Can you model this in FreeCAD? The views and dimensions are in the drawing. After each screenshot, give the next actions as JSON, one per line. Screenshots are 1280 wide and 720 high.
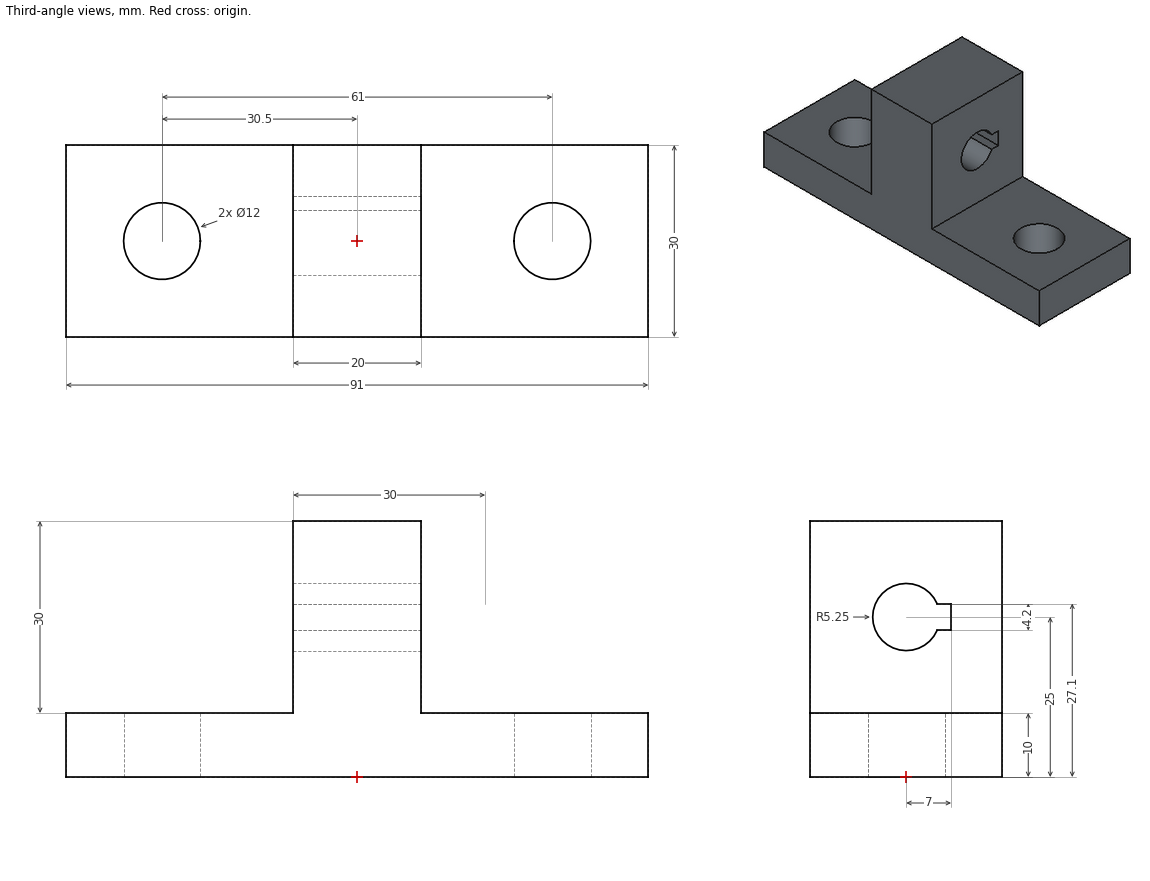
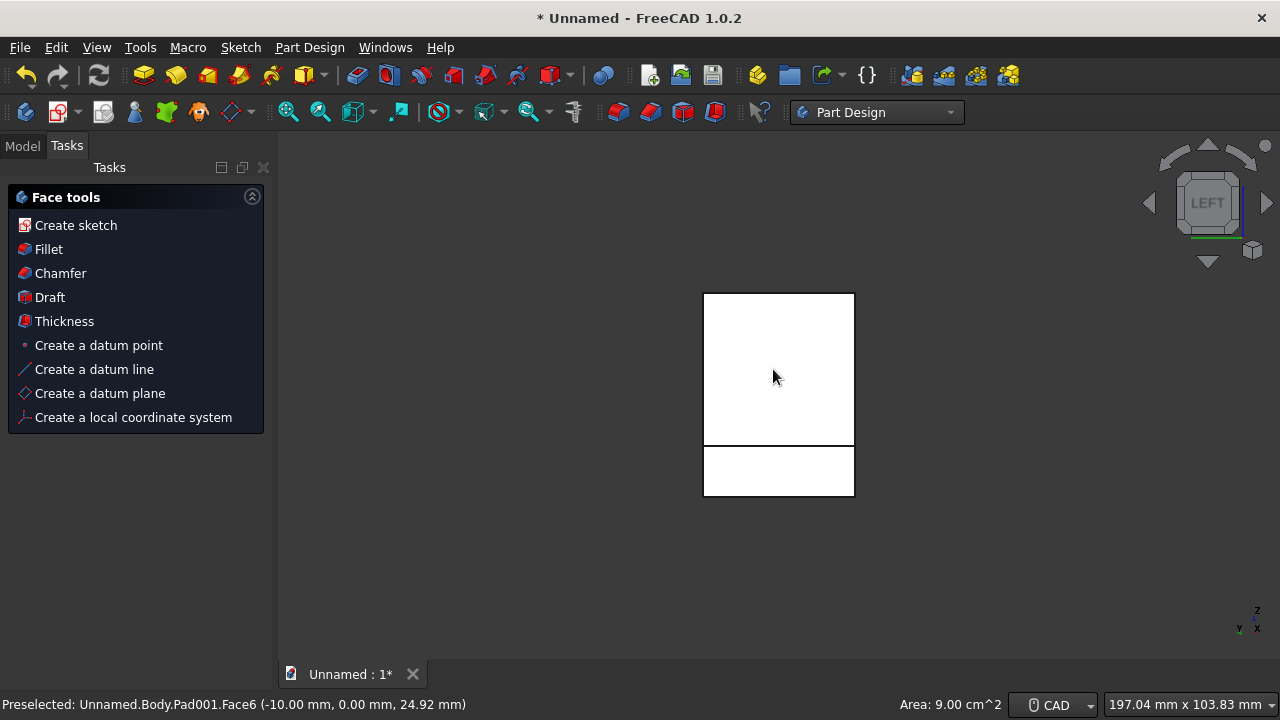
{"action": "left_click", "coordinate": [58, 112]}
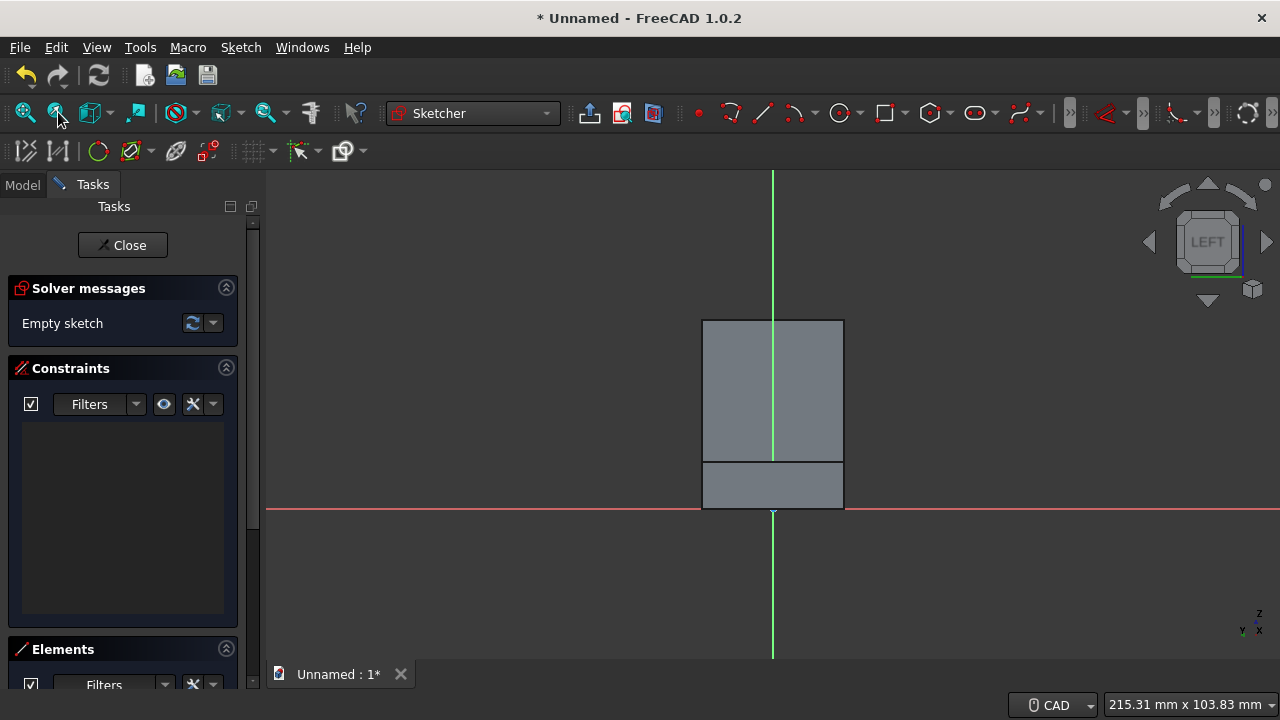
{"action": "key", "text": "q s"}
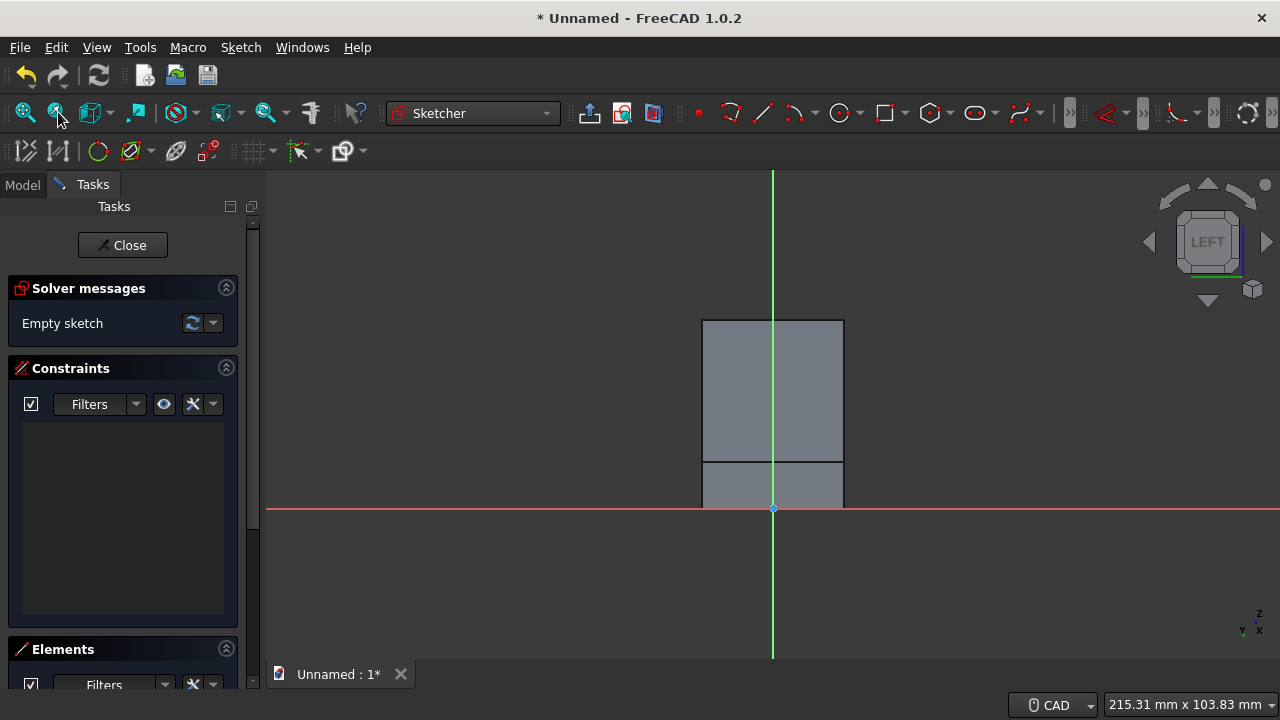
{"action": "scroll", "coordinate": [821, 470], "scroll_direction": "up", "scroll_amount": 4}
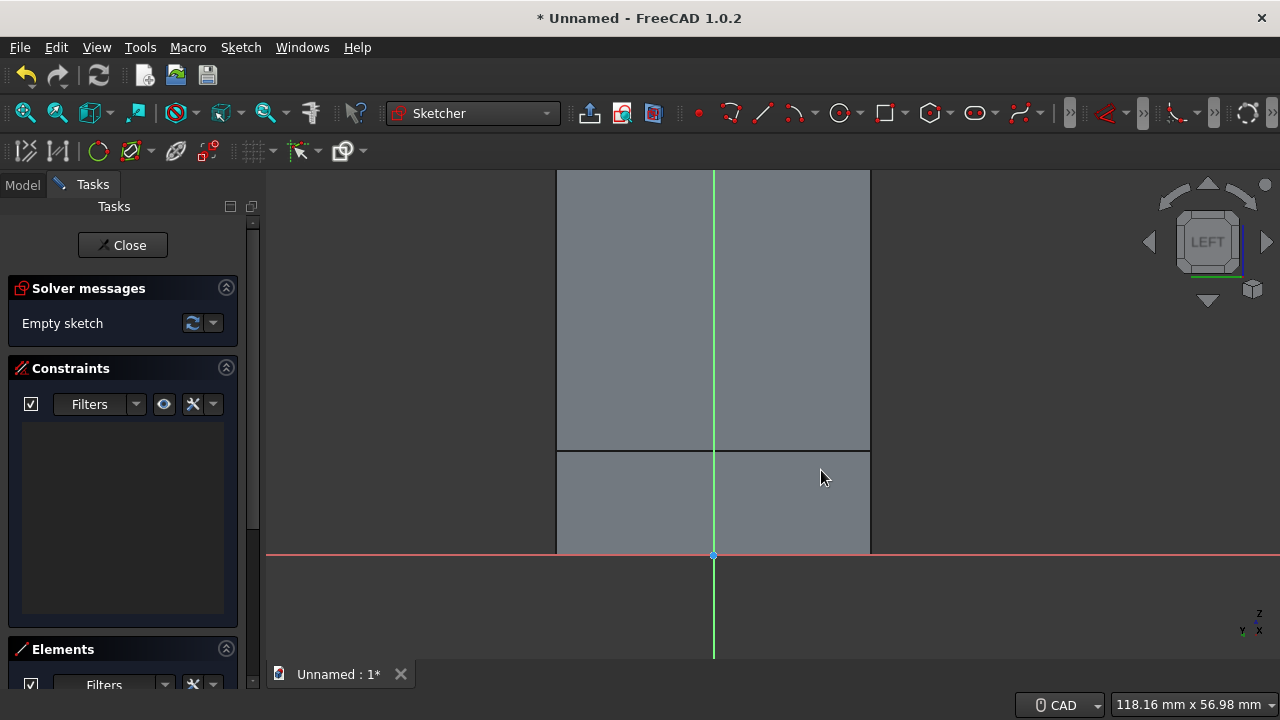
{"action": "key", "text": "g m"}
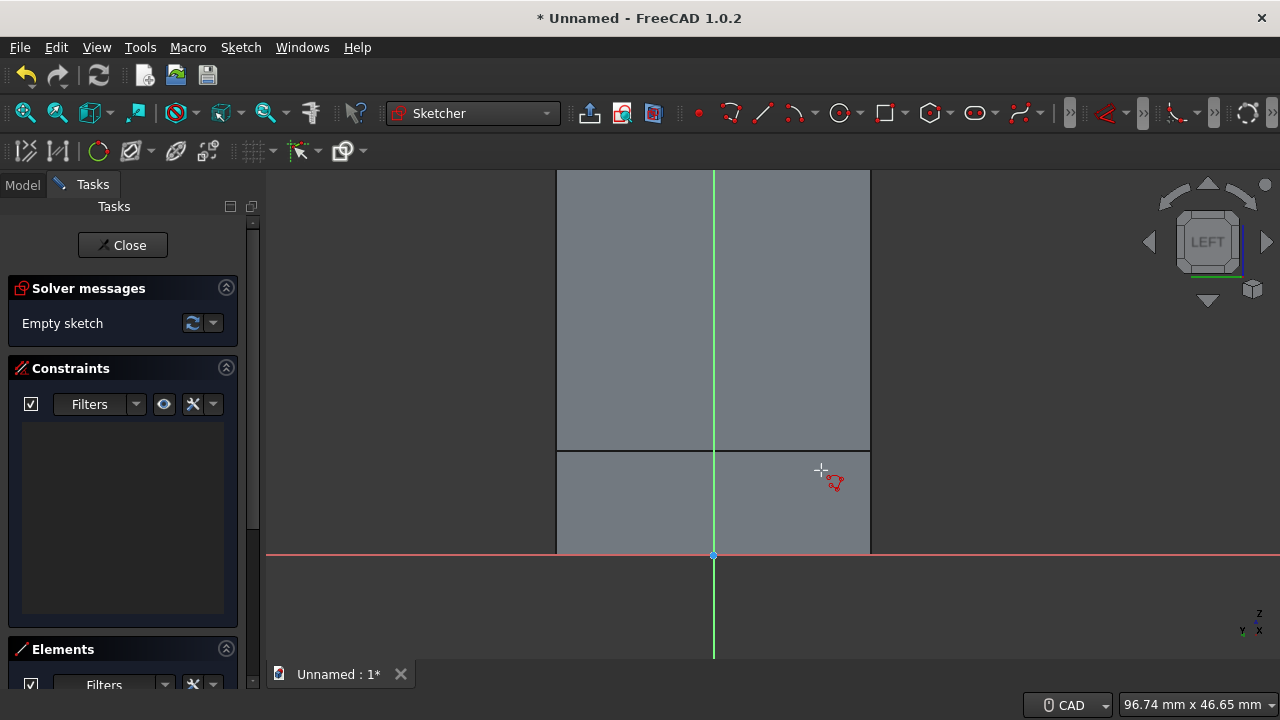
{"action": "left_click", "coordinate": [663, 271]}
{"action": "left_click", "coordinate": [640, 271]}
{"action": "left_click", "coordinate": [640, 315]}
{"action": "left_click", "coordinate": [663, 315]}
{"action": "right_click", "coordinate": [663, 315]}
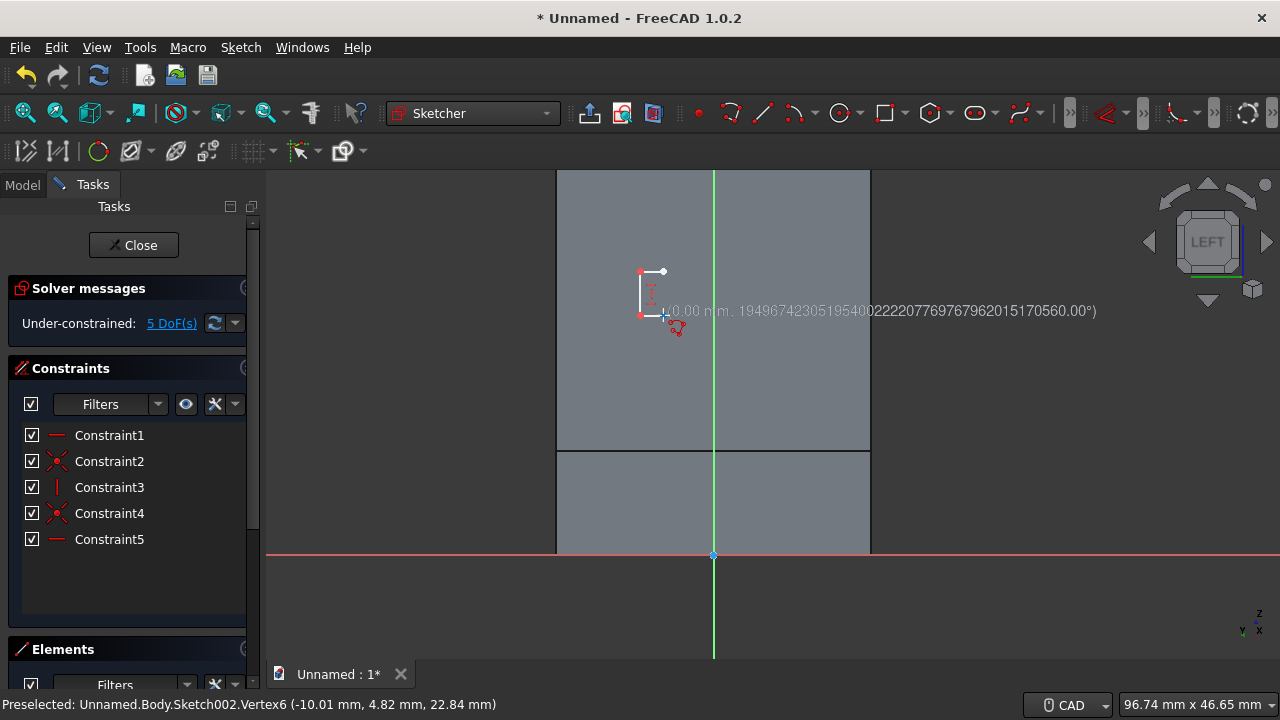
{"action": "key", "text": "g 3 a"}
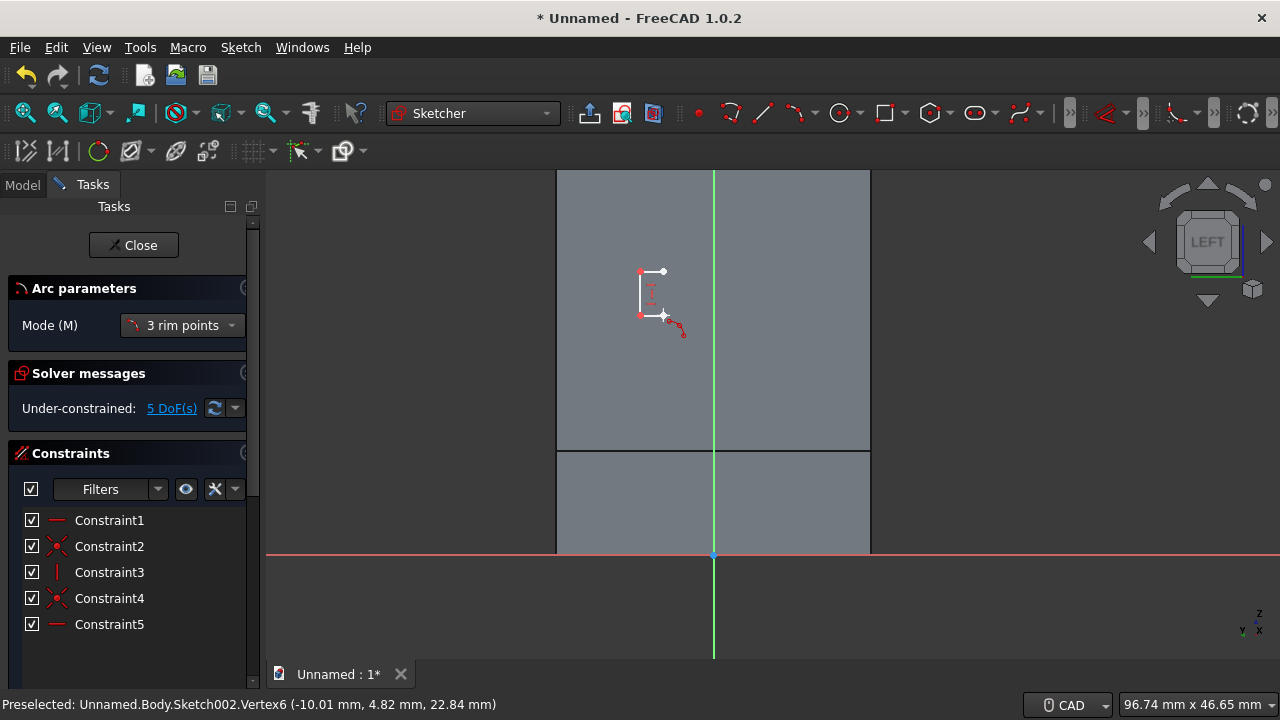
{"action": "scroll", "coordinate": [663, 315], "scroll_direction": "up", "scroll_amount": 2}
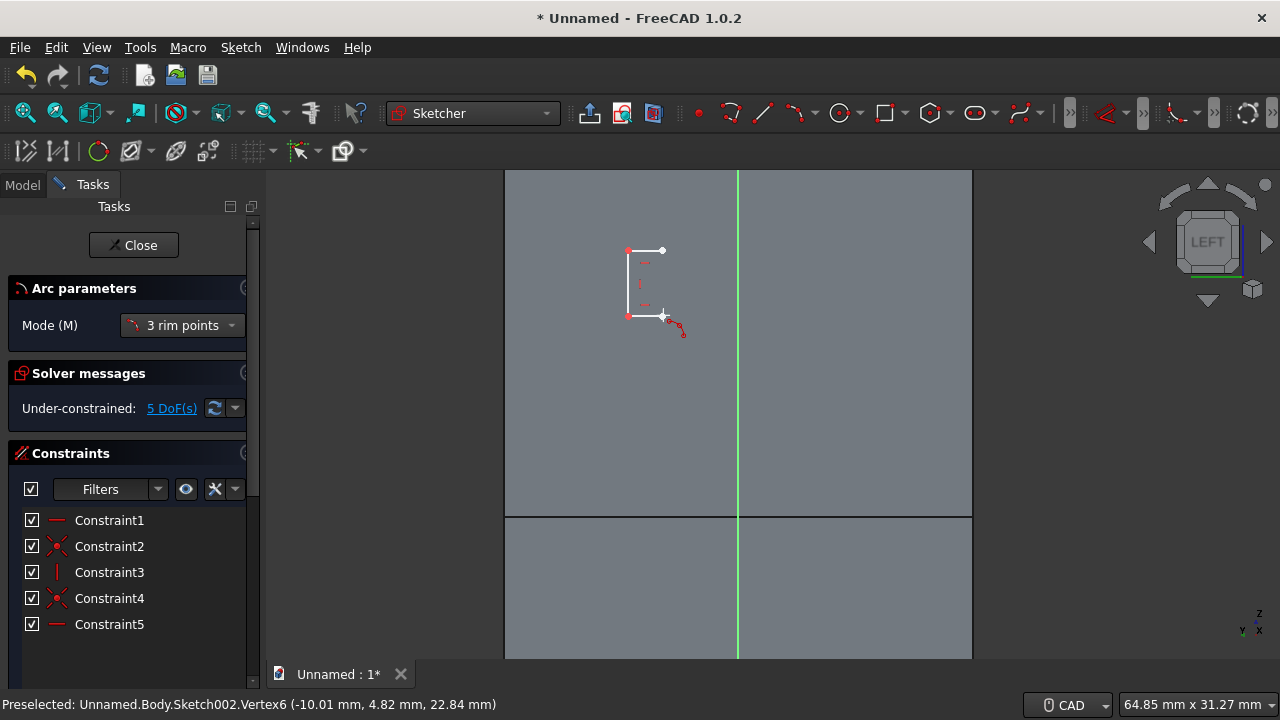
{"action": "left_click", "coordinate": [663, 316]}
{"action": "left_click", "coordinate": [663, 251]}
{"action": "left_click", "coordinate": [820, 283]}
{"action": "key", "text": "Escape"}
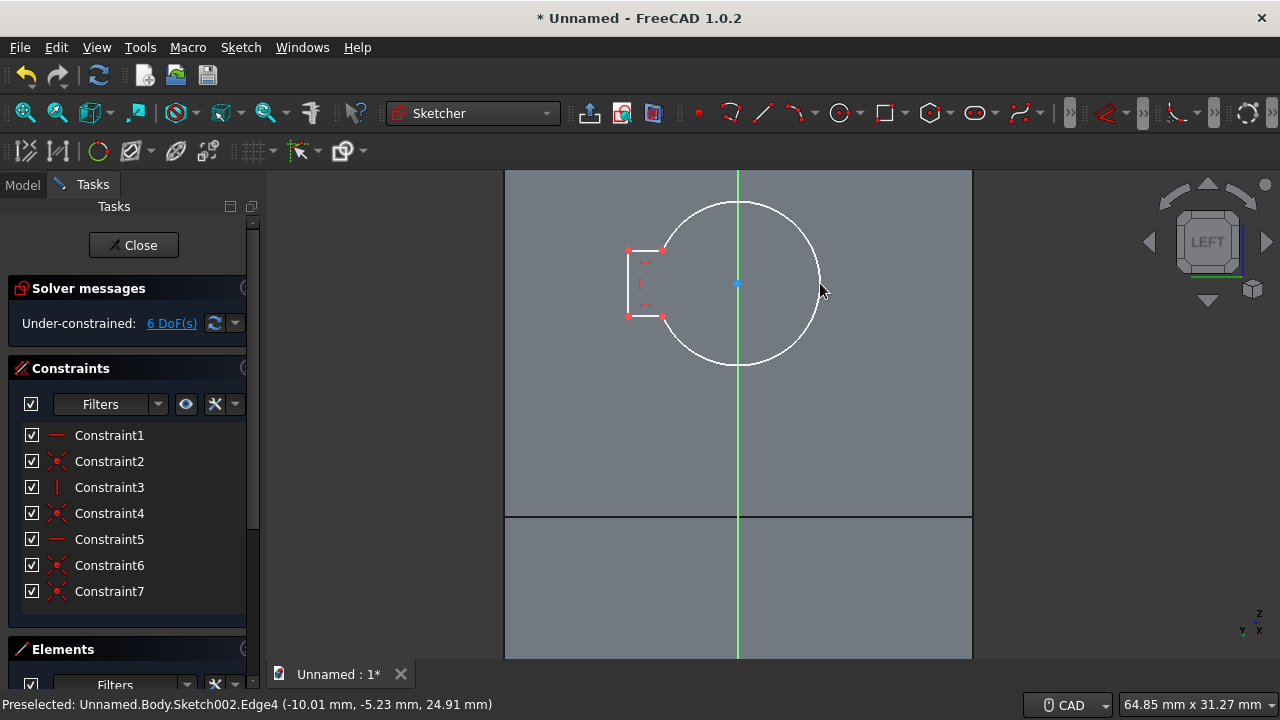
{"action": "left_click", "coordinate": [738, 284]}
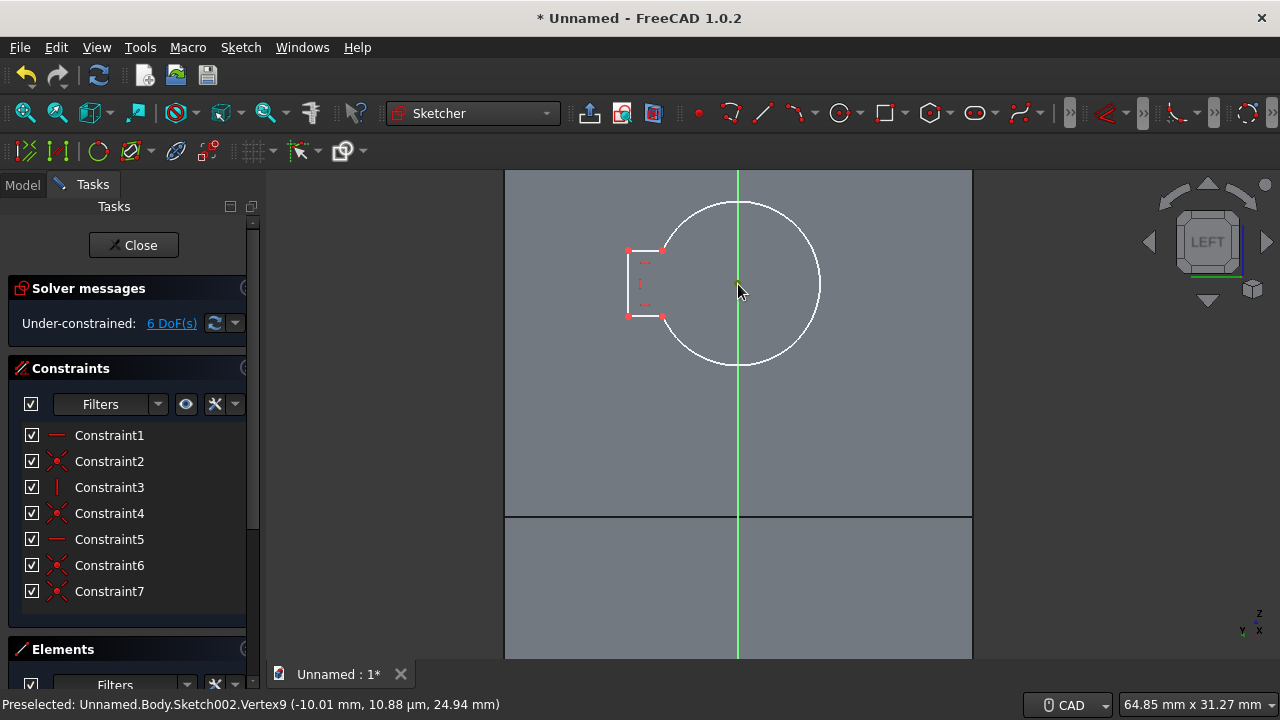
{"action": "left_click", "coordinate": [738, 600]}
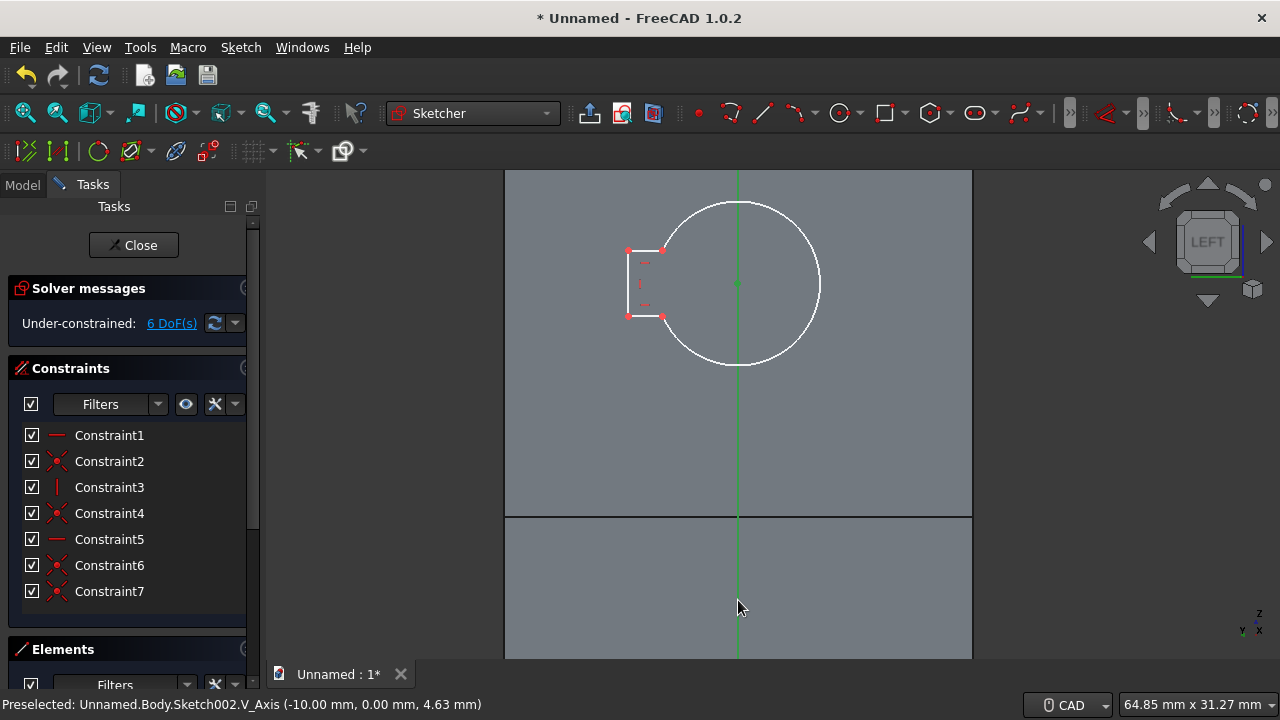
{"action": "key", "text": "c"}